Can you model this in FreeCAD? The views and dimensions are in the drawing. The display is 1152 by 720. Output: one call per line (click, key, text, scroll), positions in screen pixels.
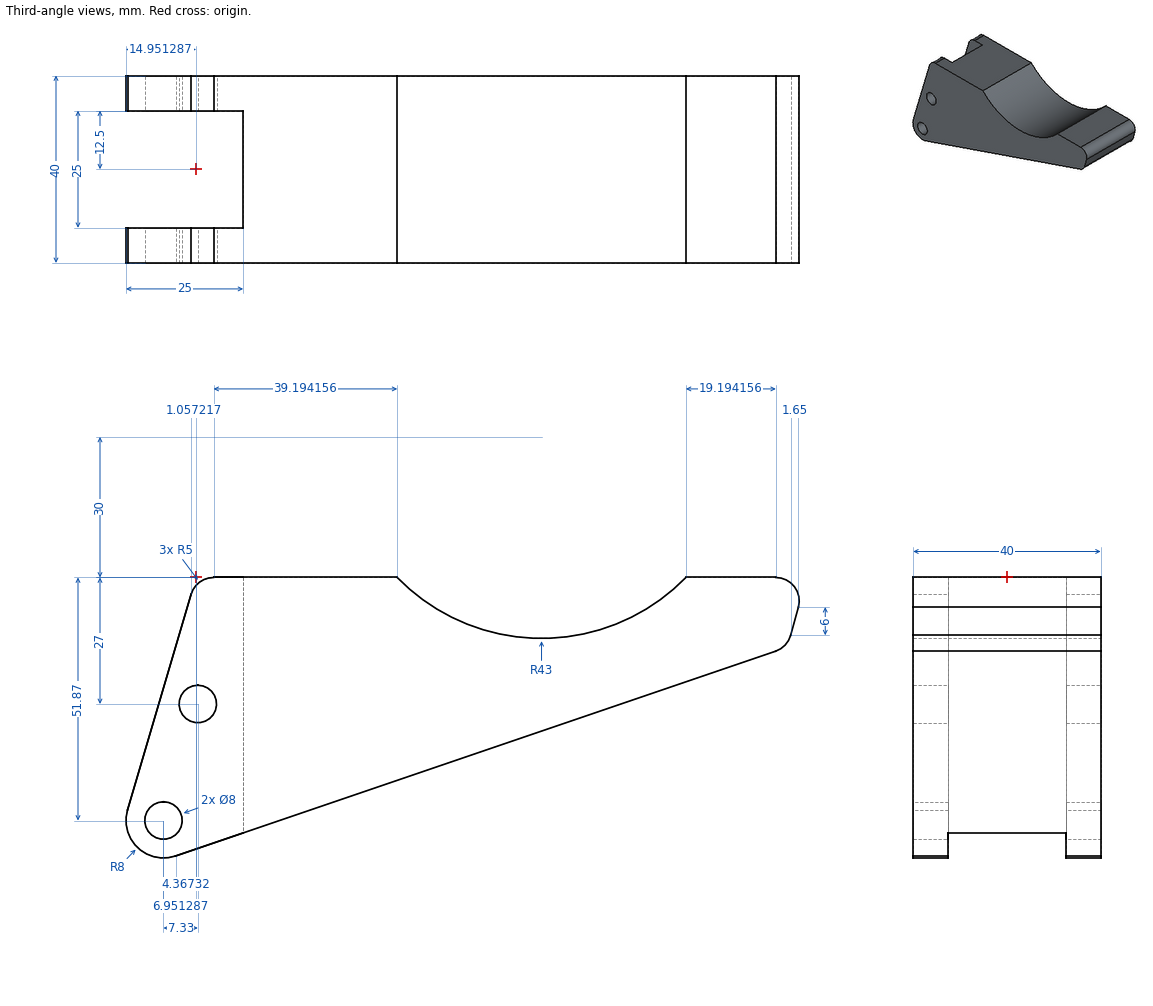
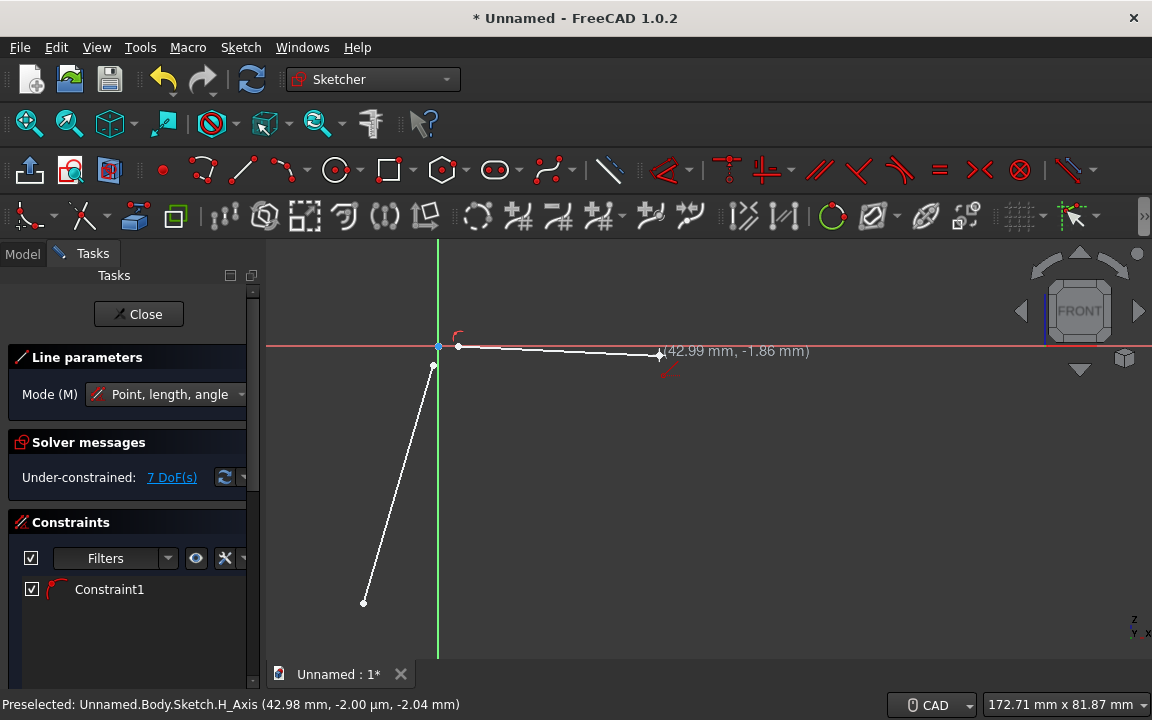
click(975, 346)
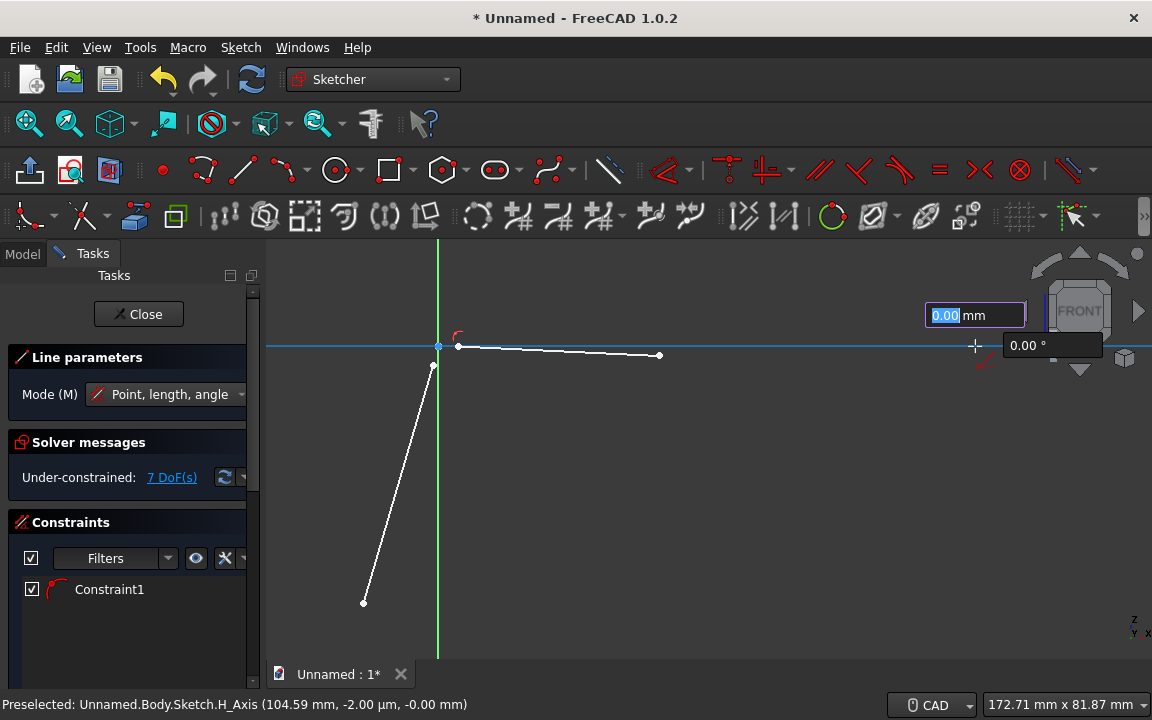
scroll(457, 347, down, 2)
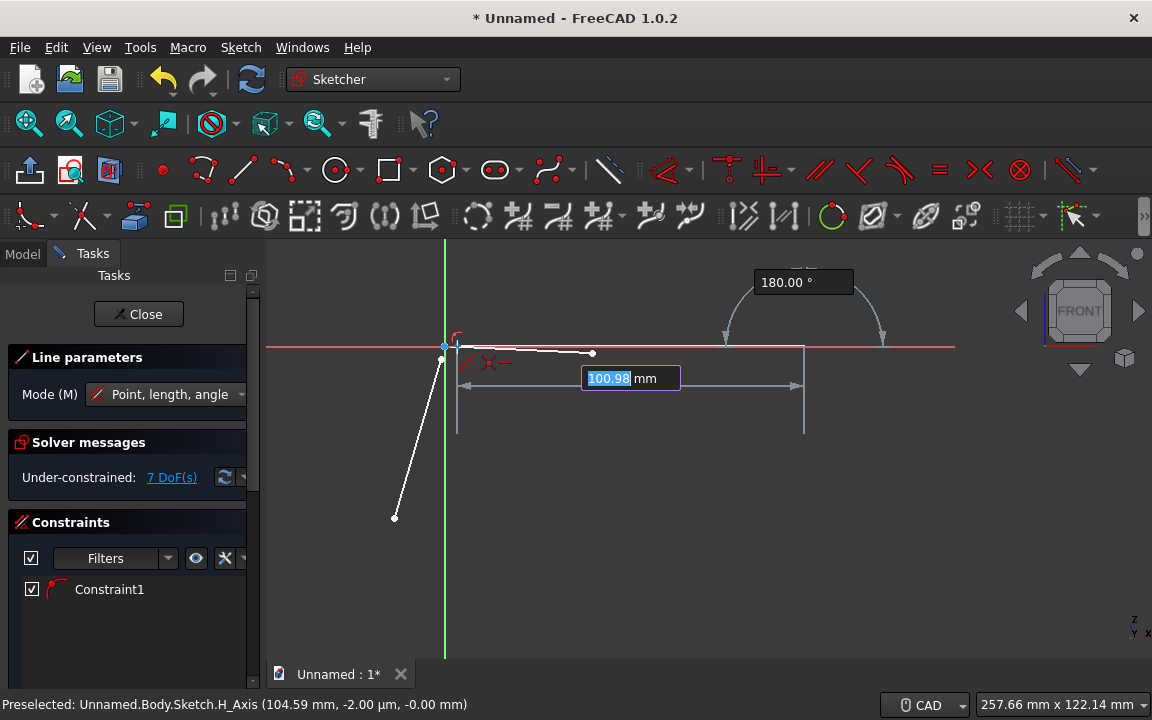
click(870, 356)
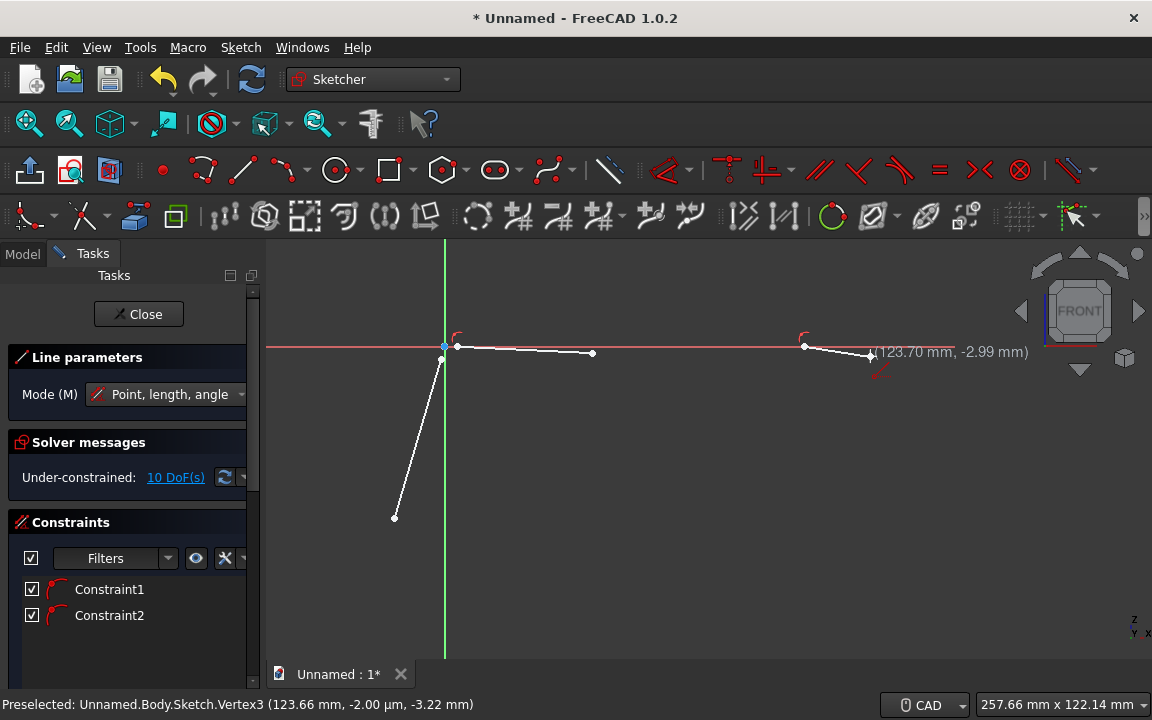
click(887, 368)
click(881, 389)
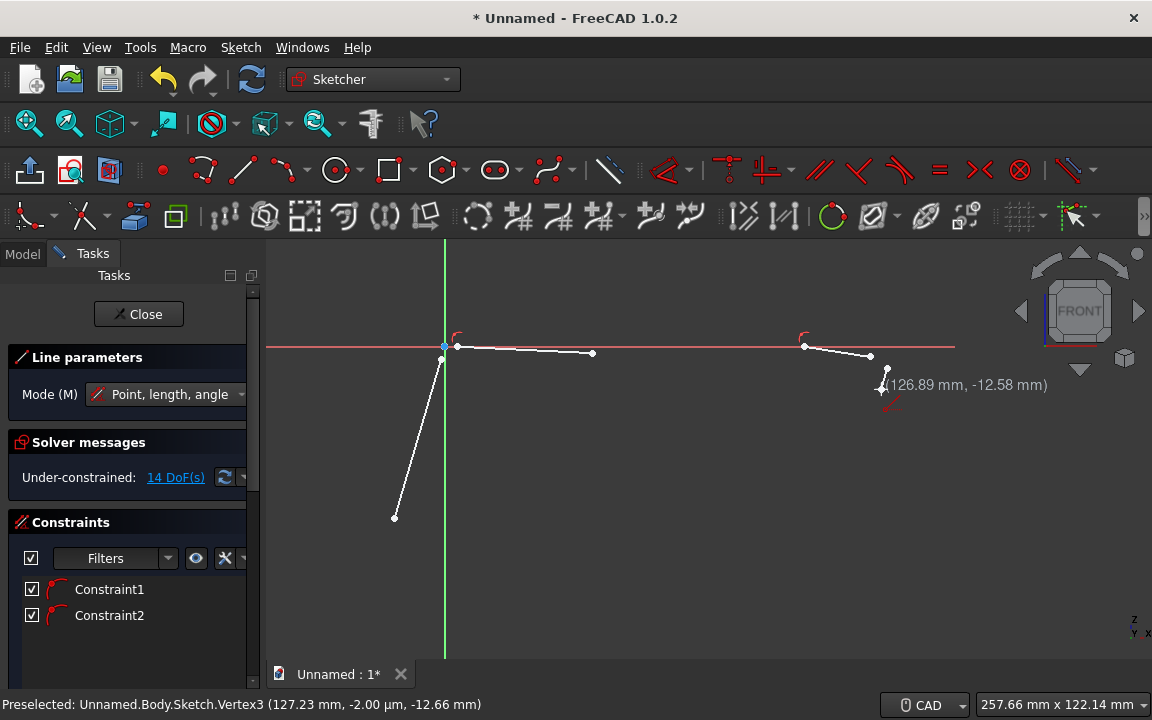
click(870, 401)
click(430, 551)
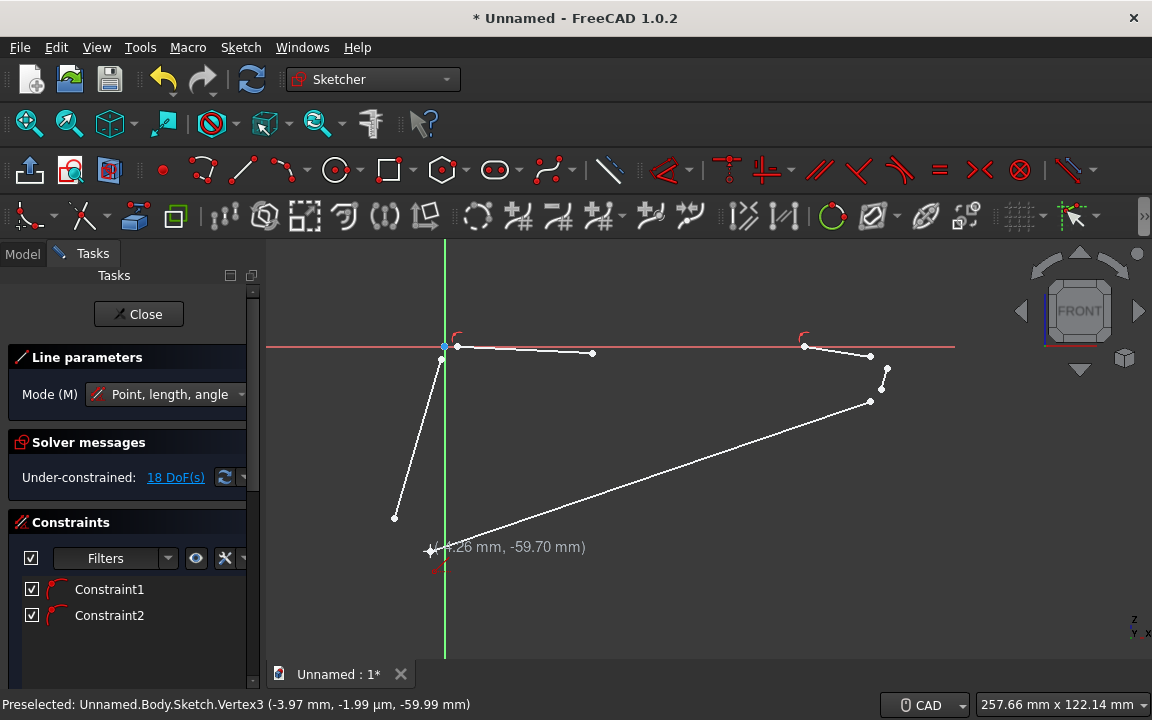
click(284, 170)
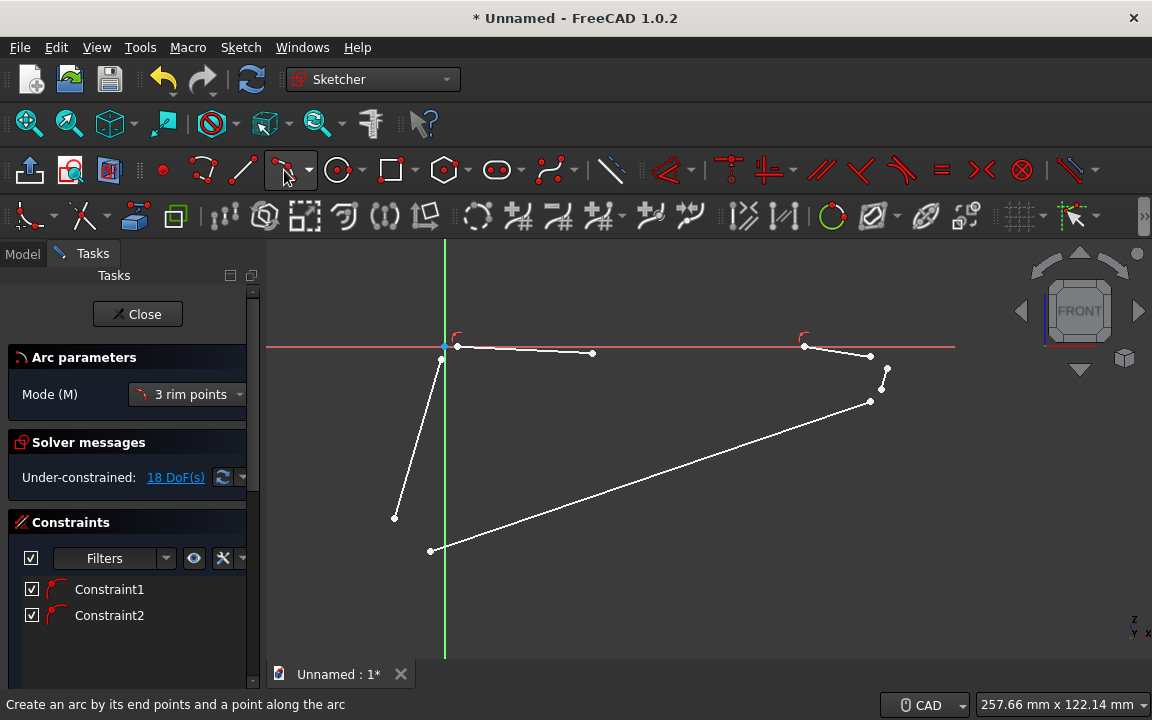
scroll(441, 359, up, 8)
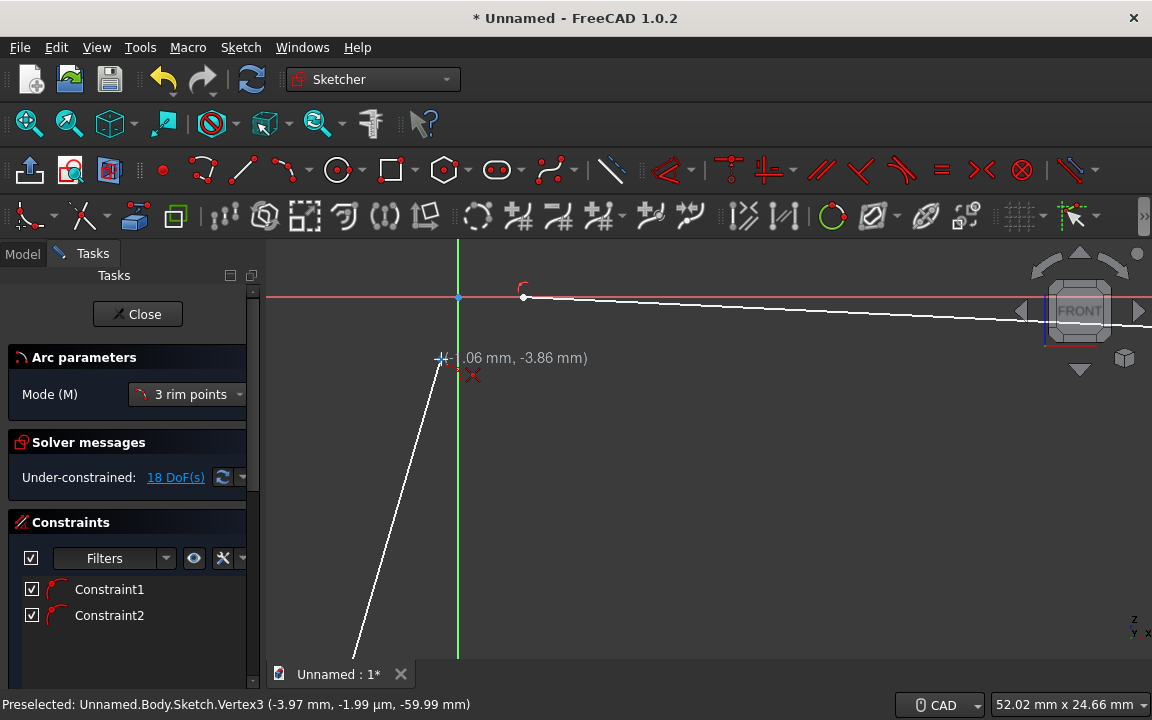
click(441, 359)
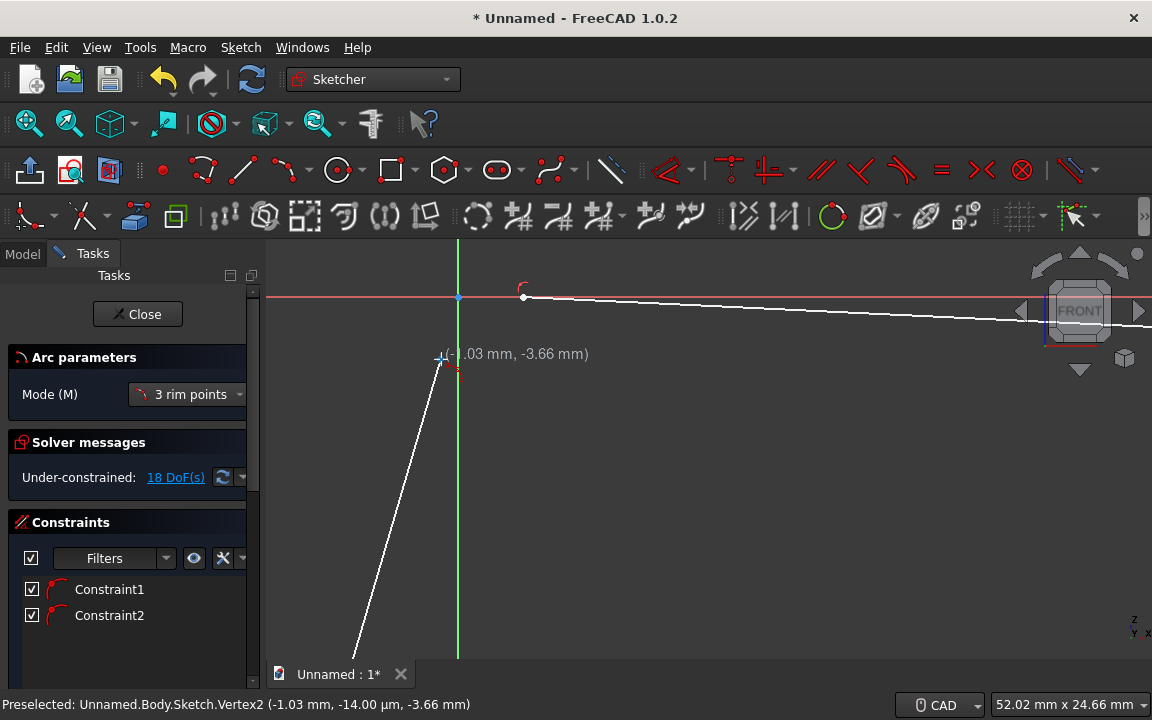
scroll(441, 359, down, 8)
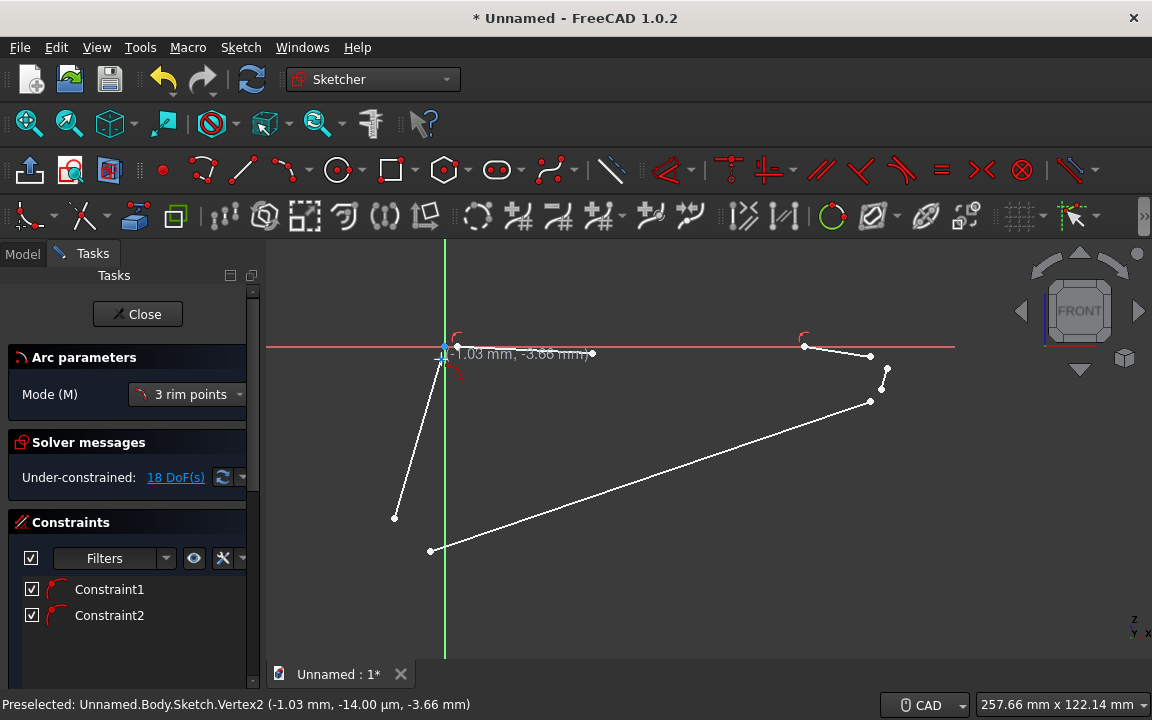
scroll(458, 347, up, 2)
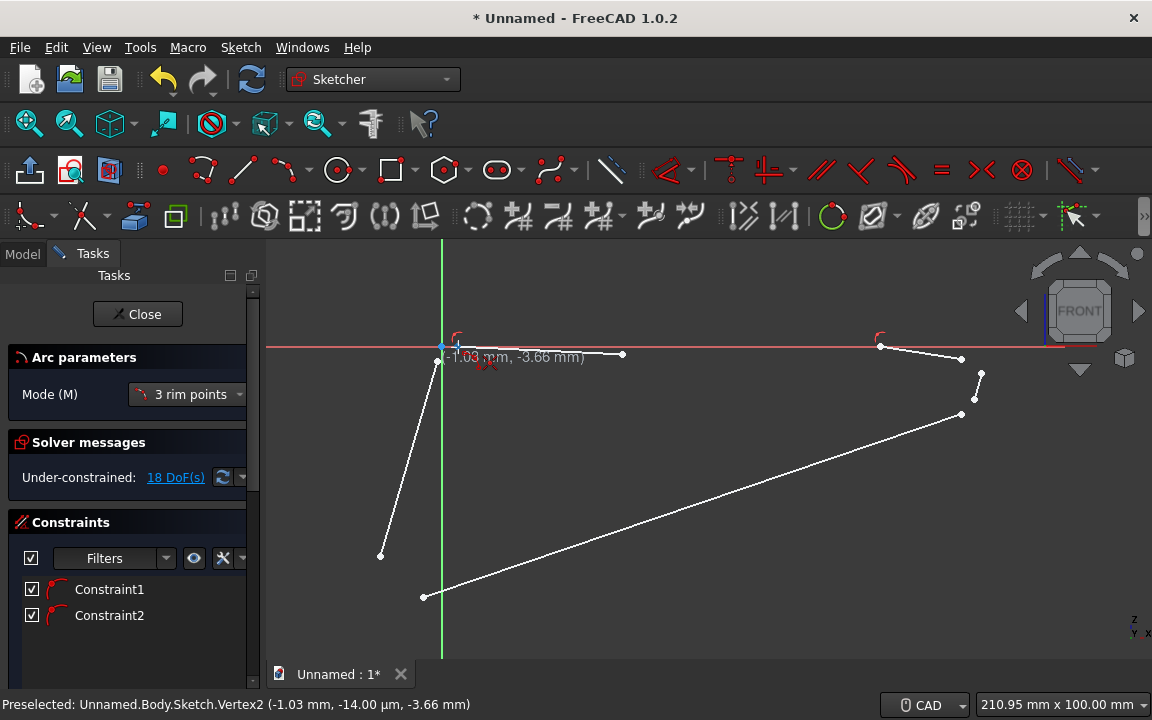
click(458, 346)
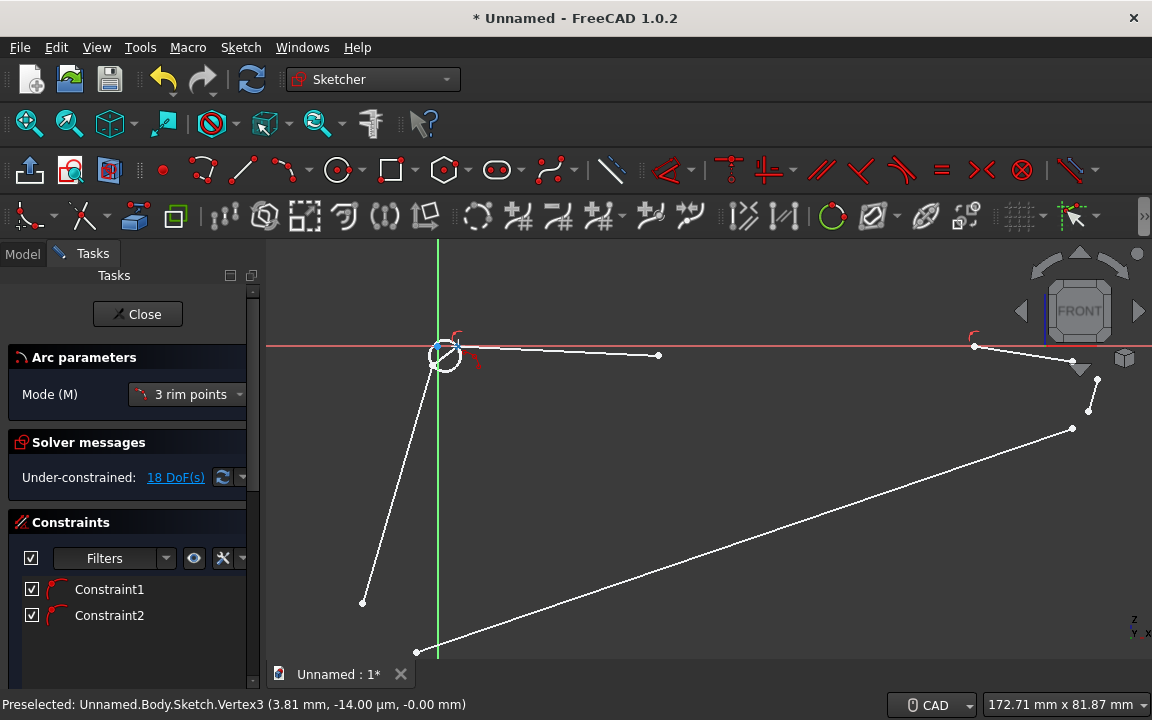
scroll(442, 352, up, 8)